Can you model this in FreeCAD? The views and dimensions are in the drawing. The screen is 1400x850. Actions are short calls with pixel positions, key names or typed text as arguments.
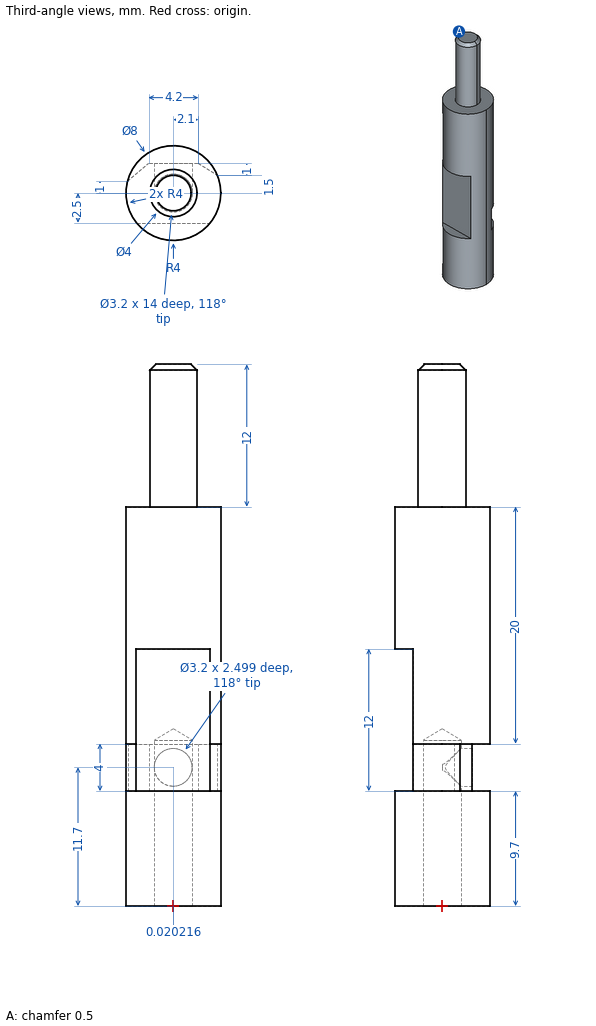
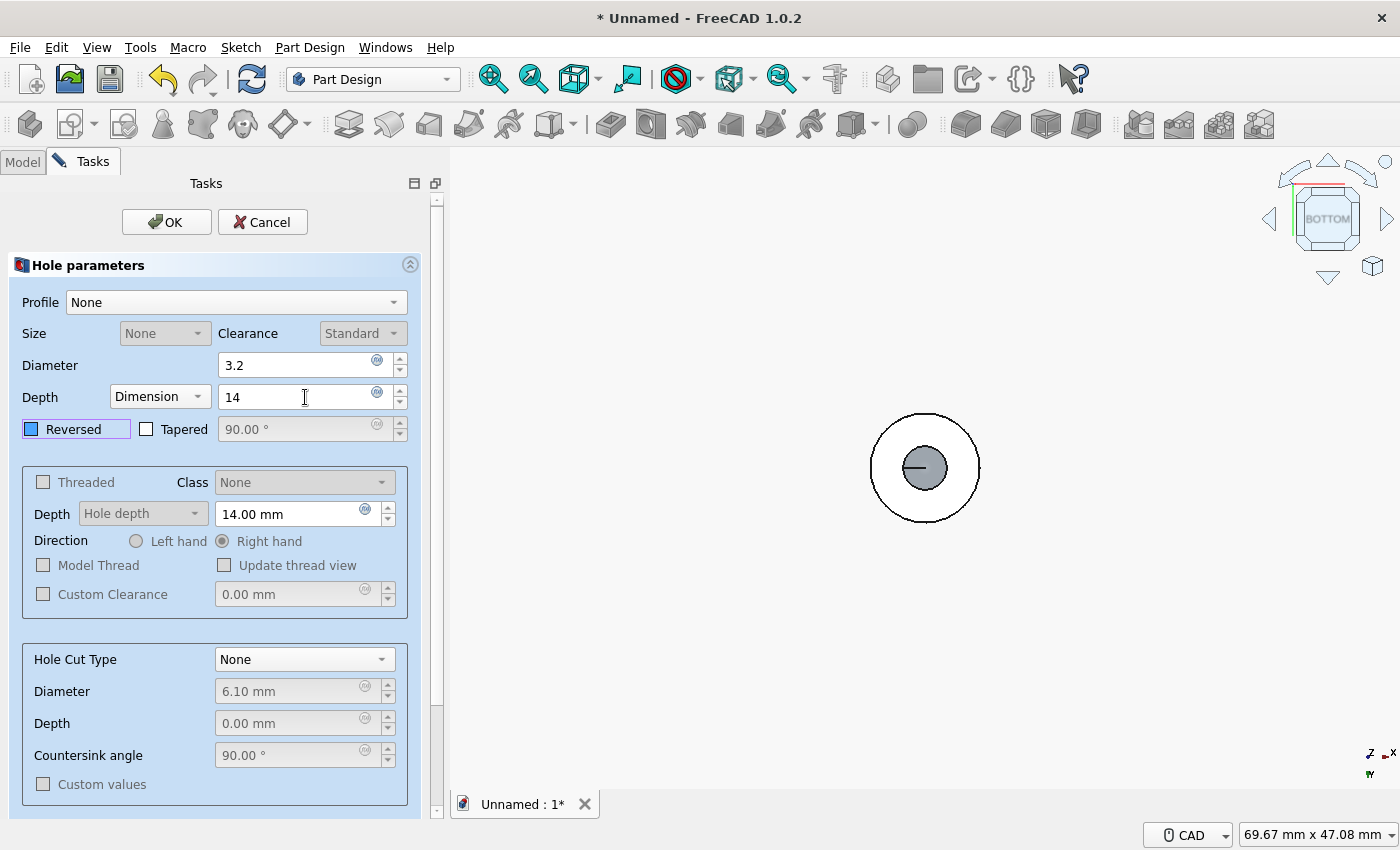
click(167, 222)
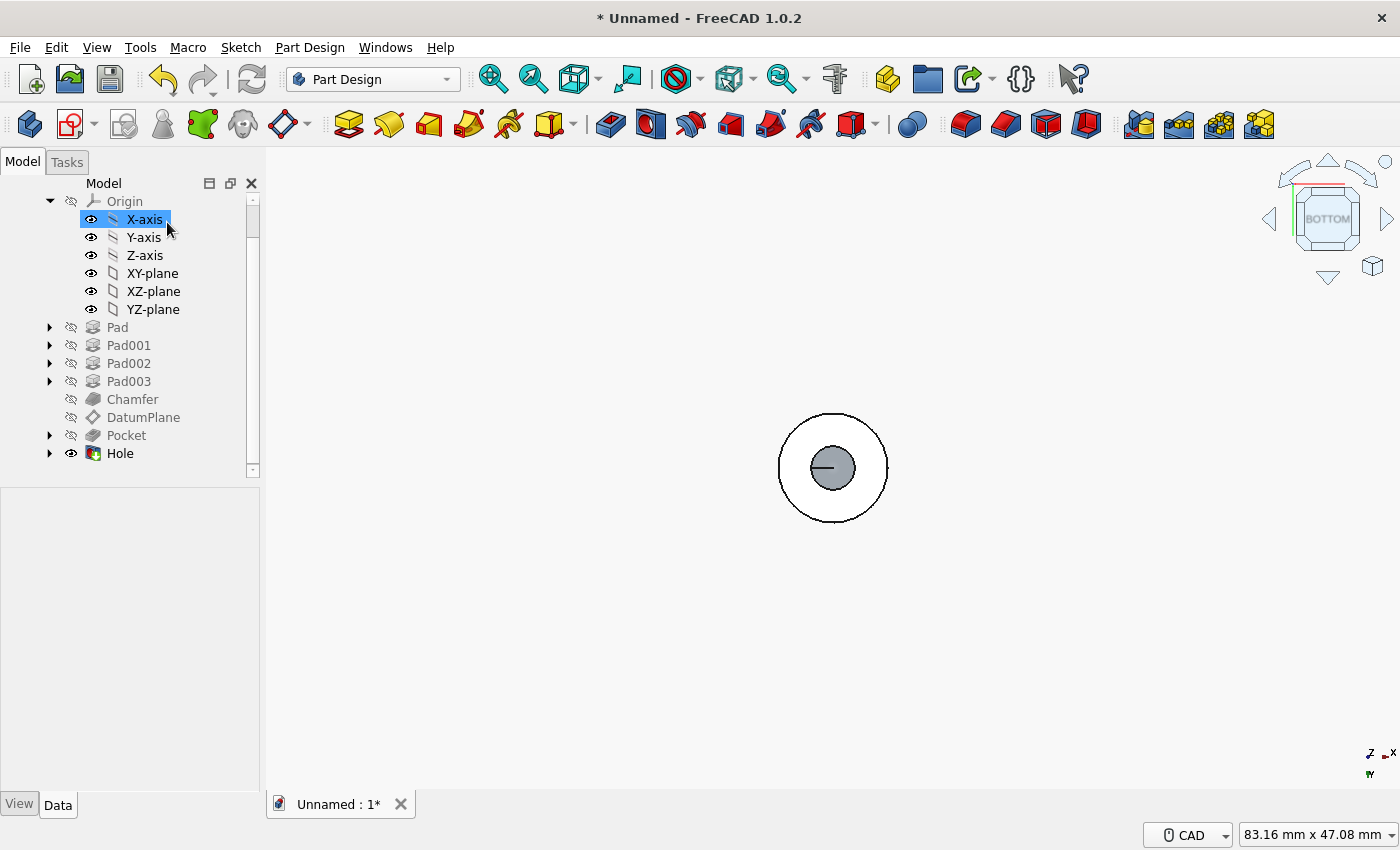
click(494, 80)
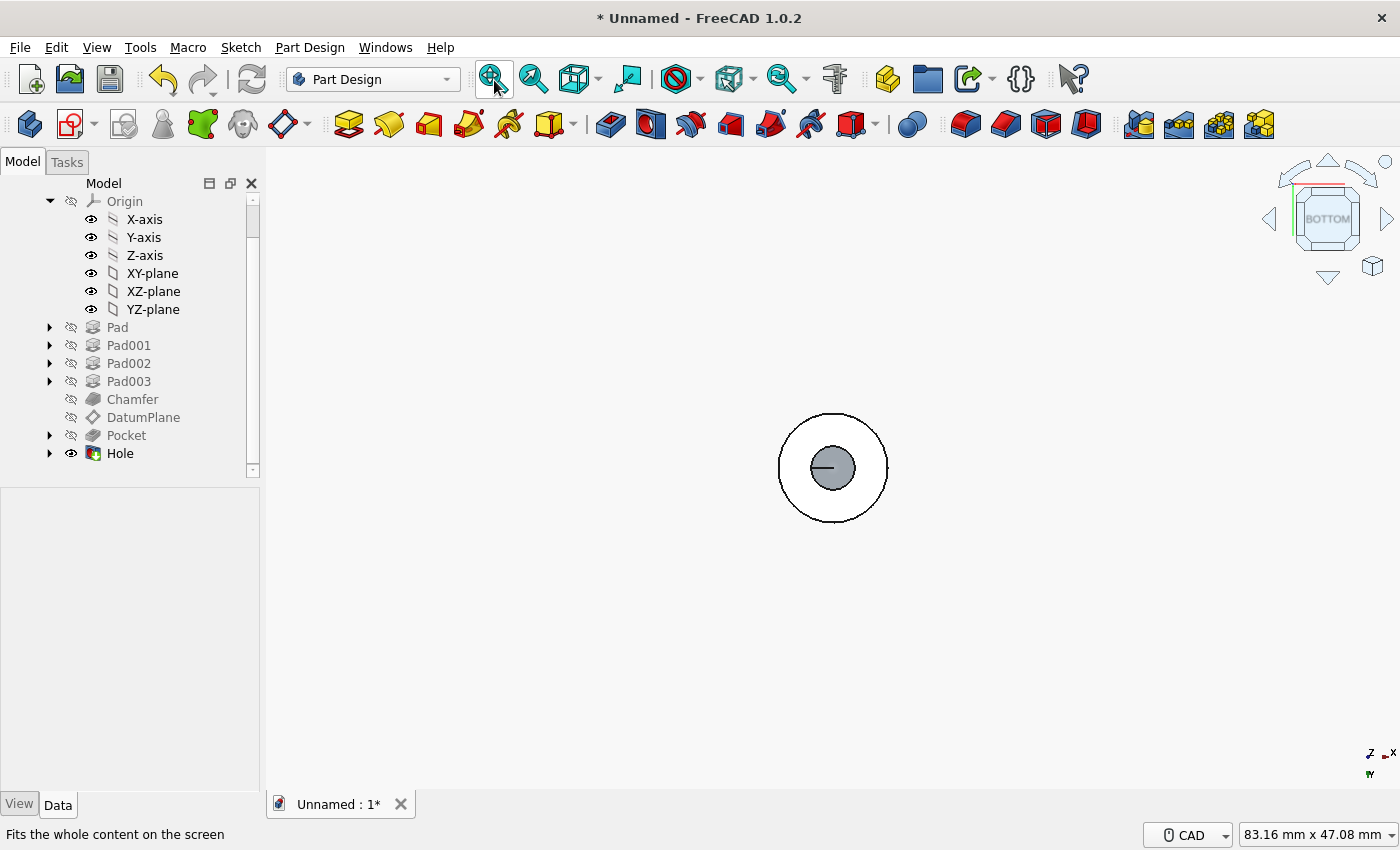
key(4)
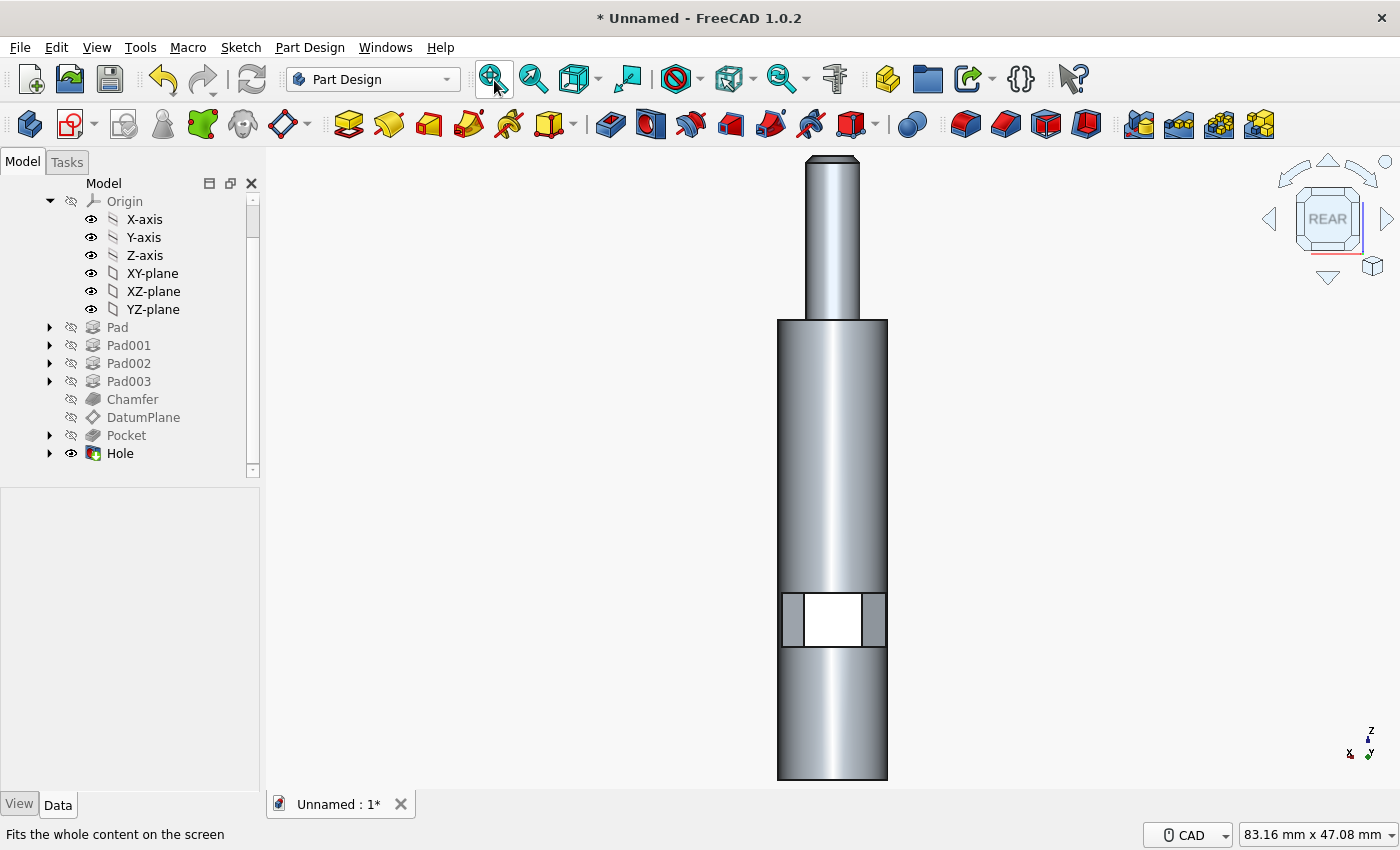
click(833, 619)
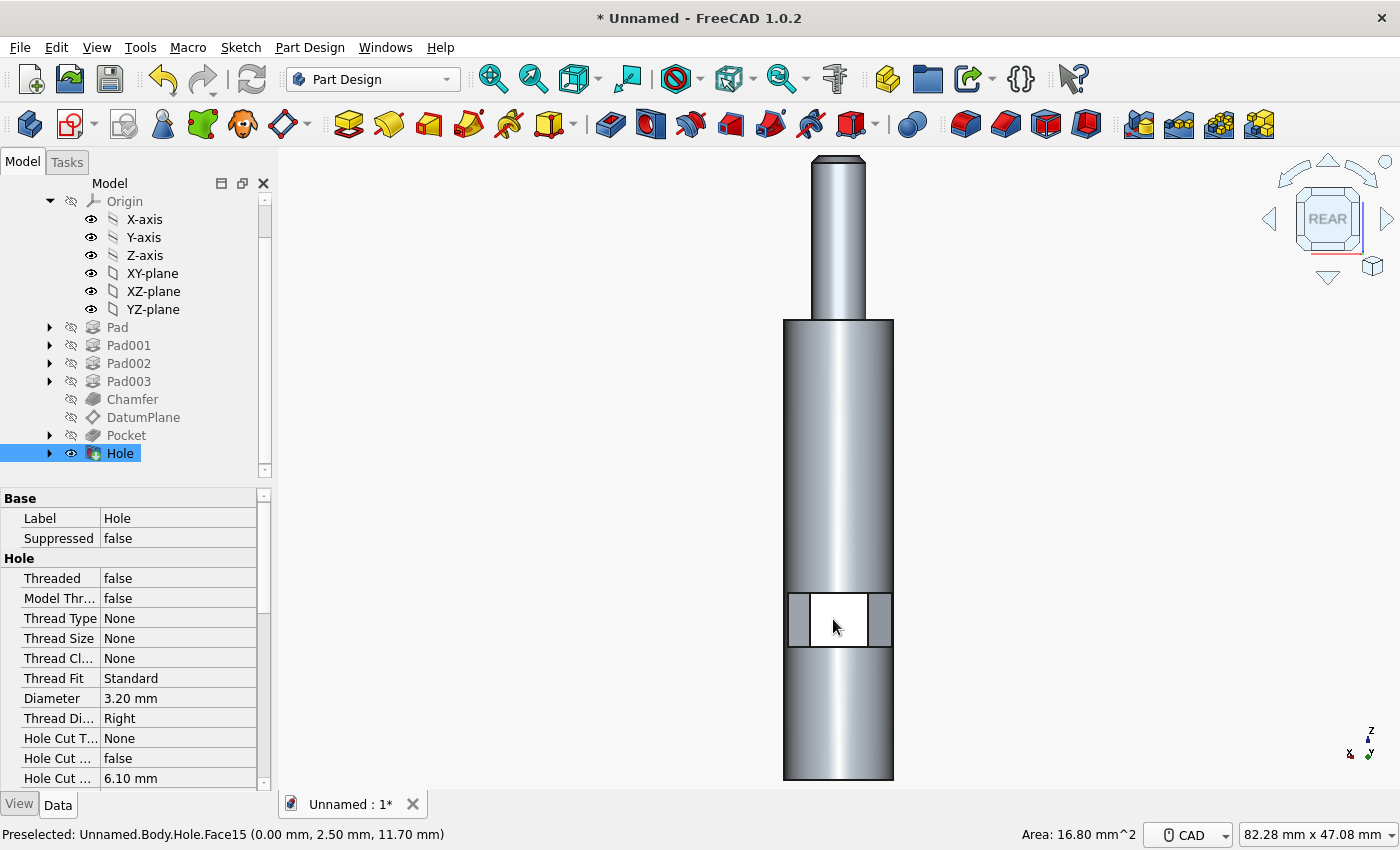
click(70, 124)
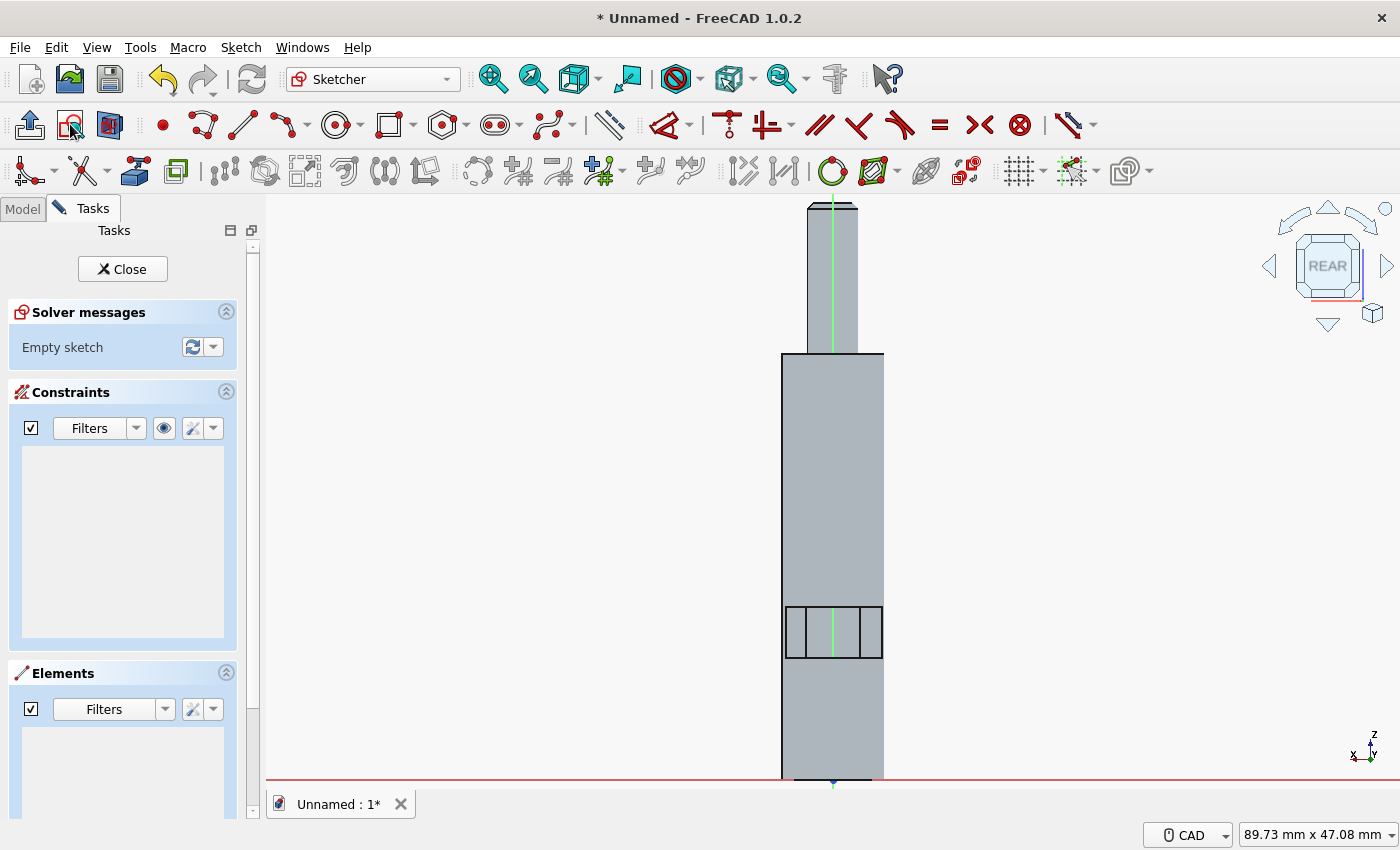
scroll(842, 650, up, 11)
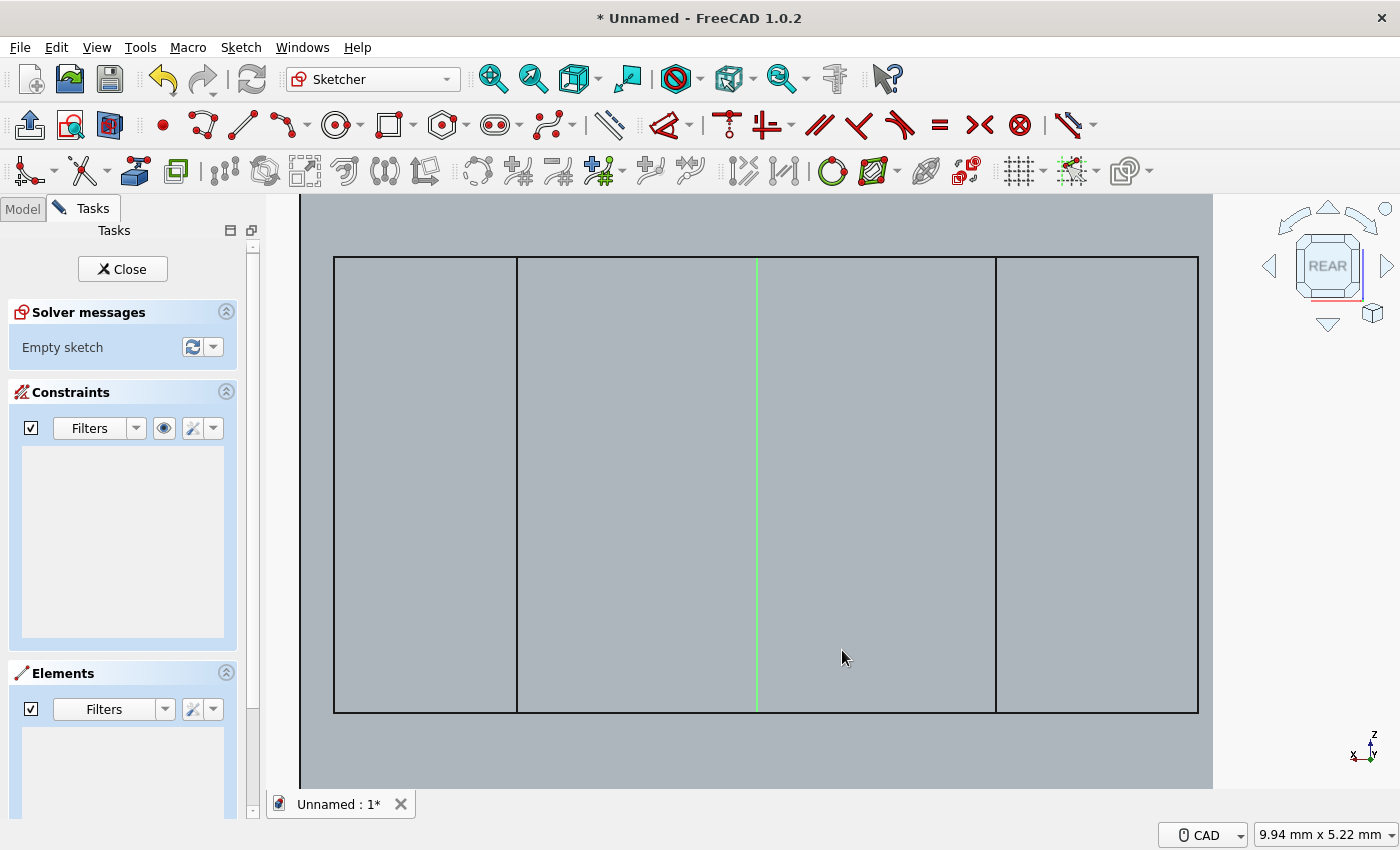
click(336, 126)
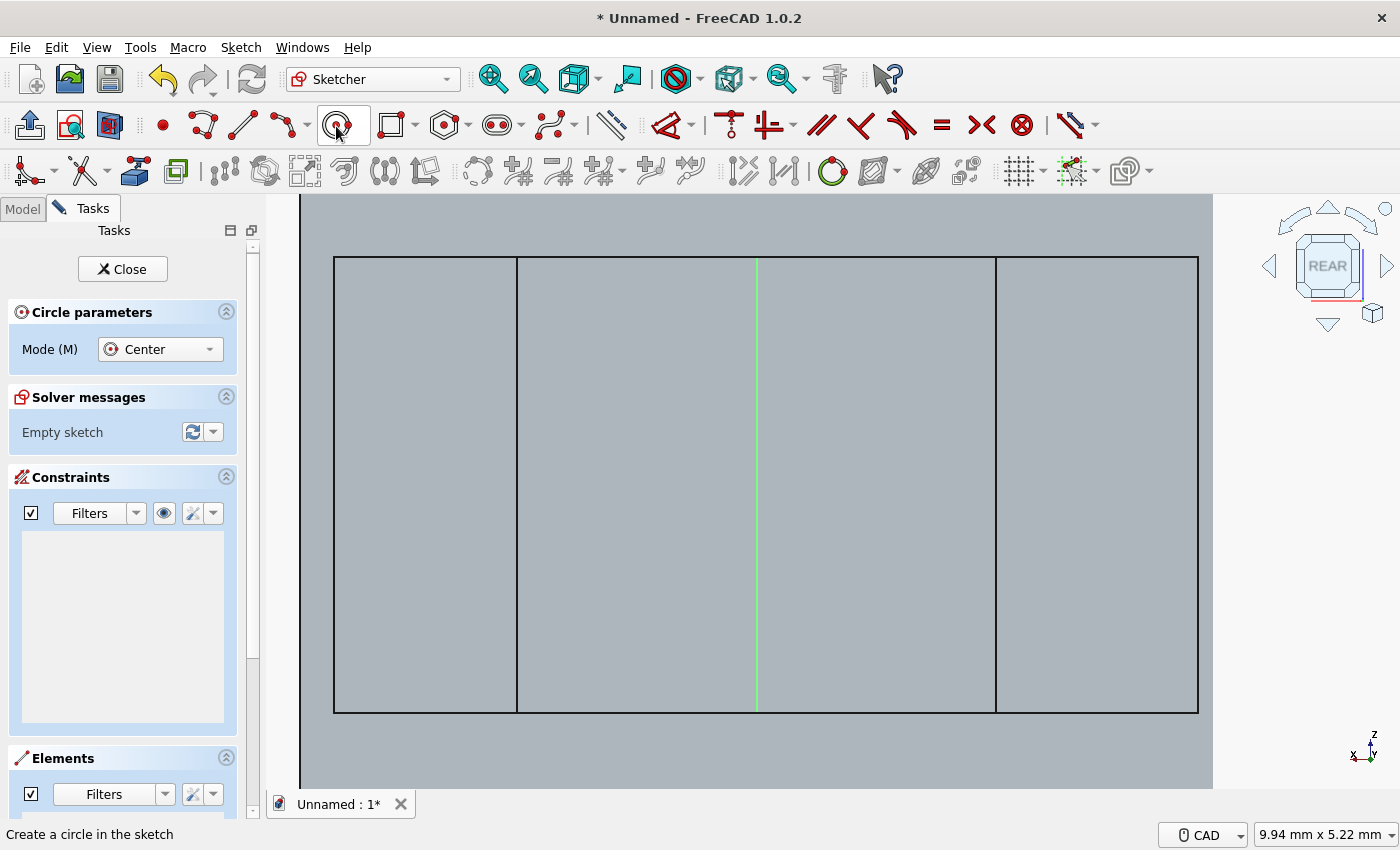
scroll(759, 485, up, 10)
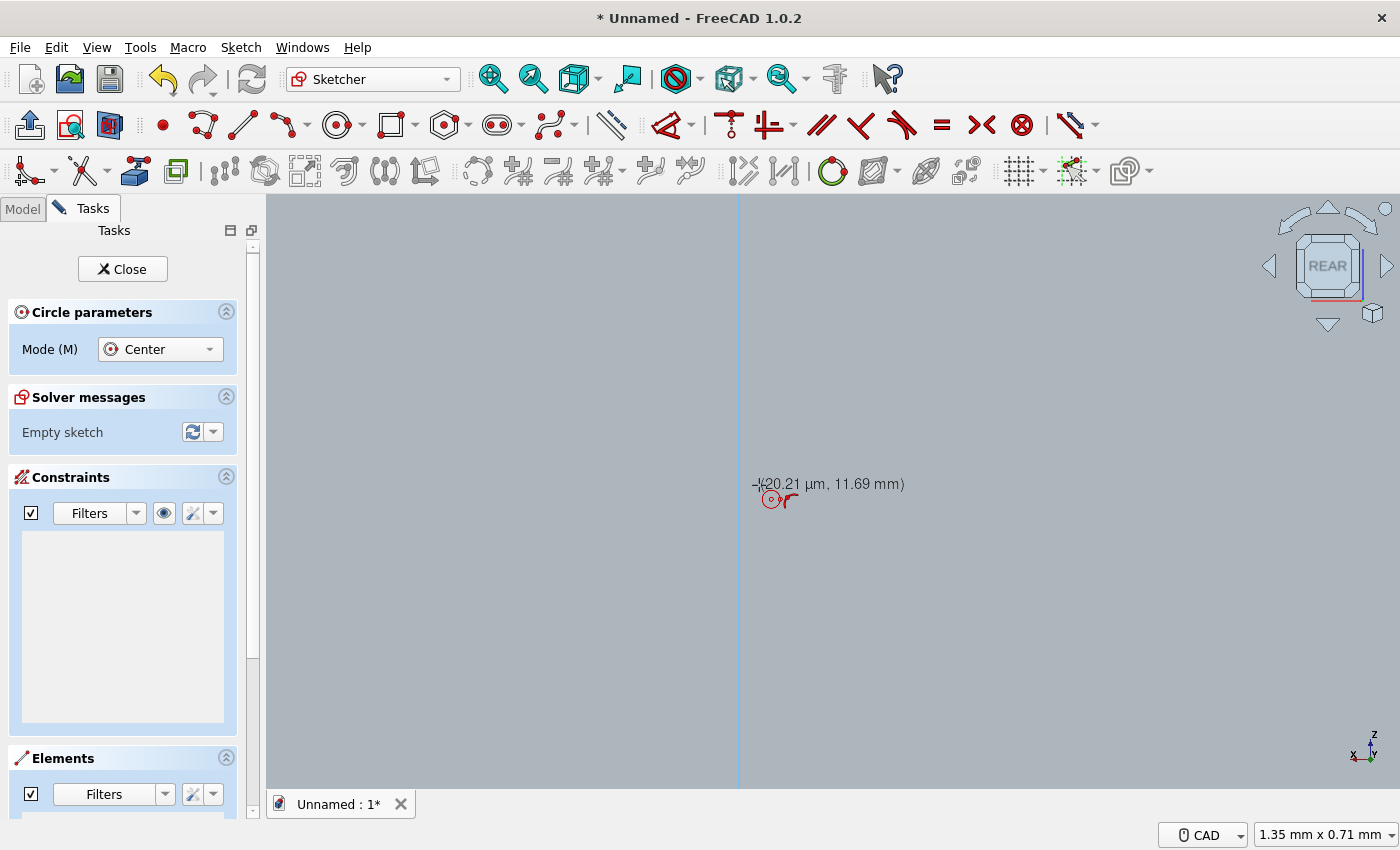
click(756, 483)